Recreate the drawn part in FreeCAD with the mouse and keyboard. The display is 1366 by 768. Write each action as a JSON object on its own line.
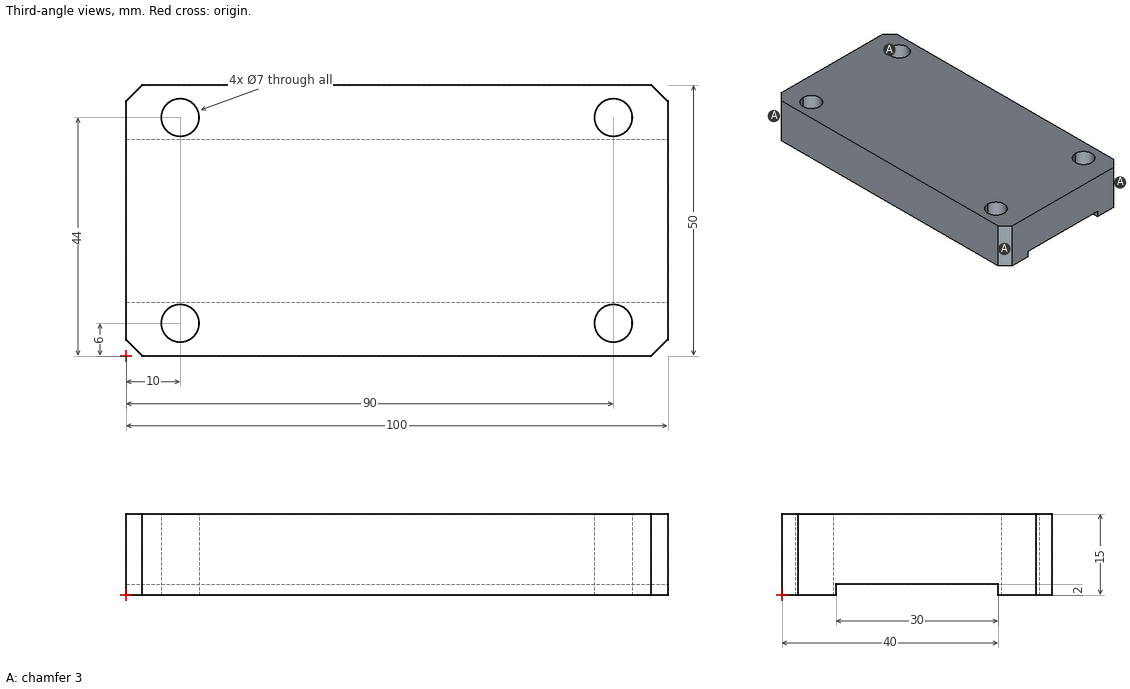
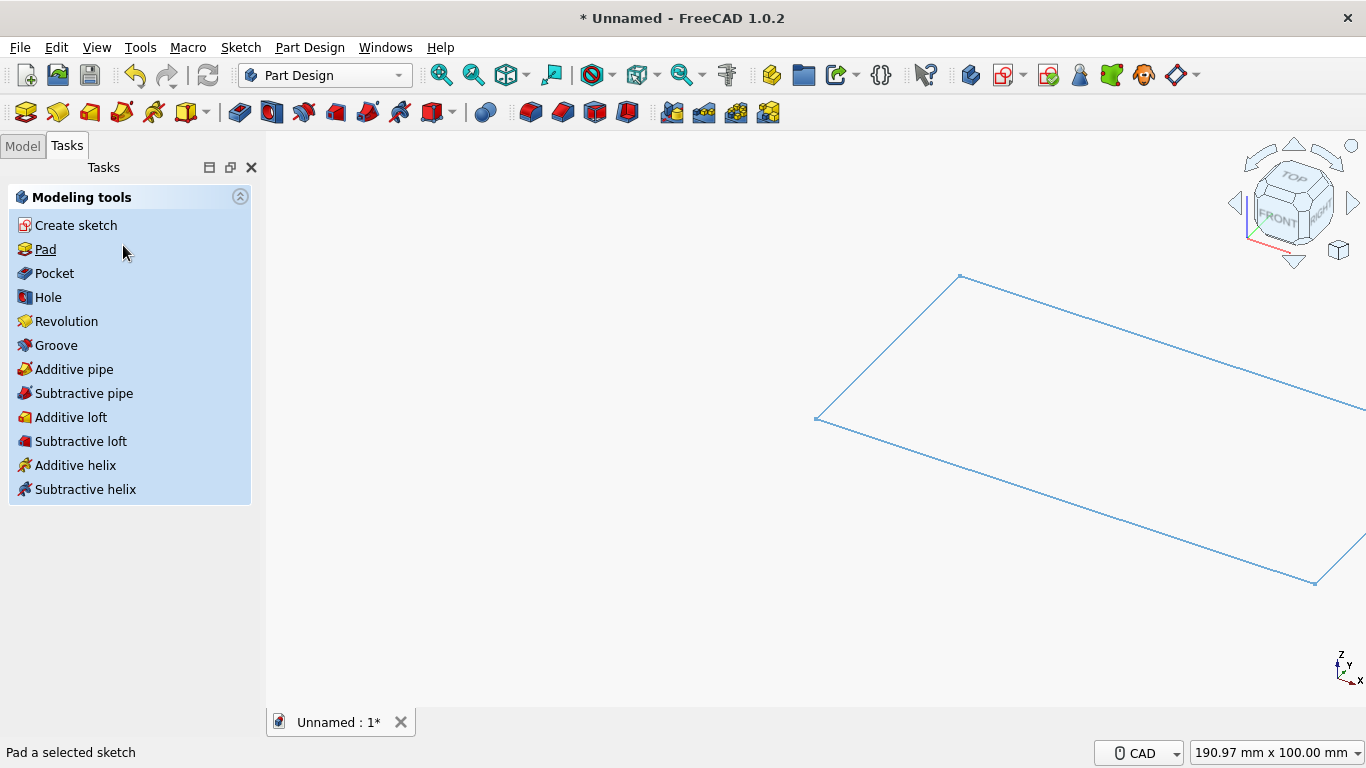
{"action": "left_click", "coordinate": [26, 112]}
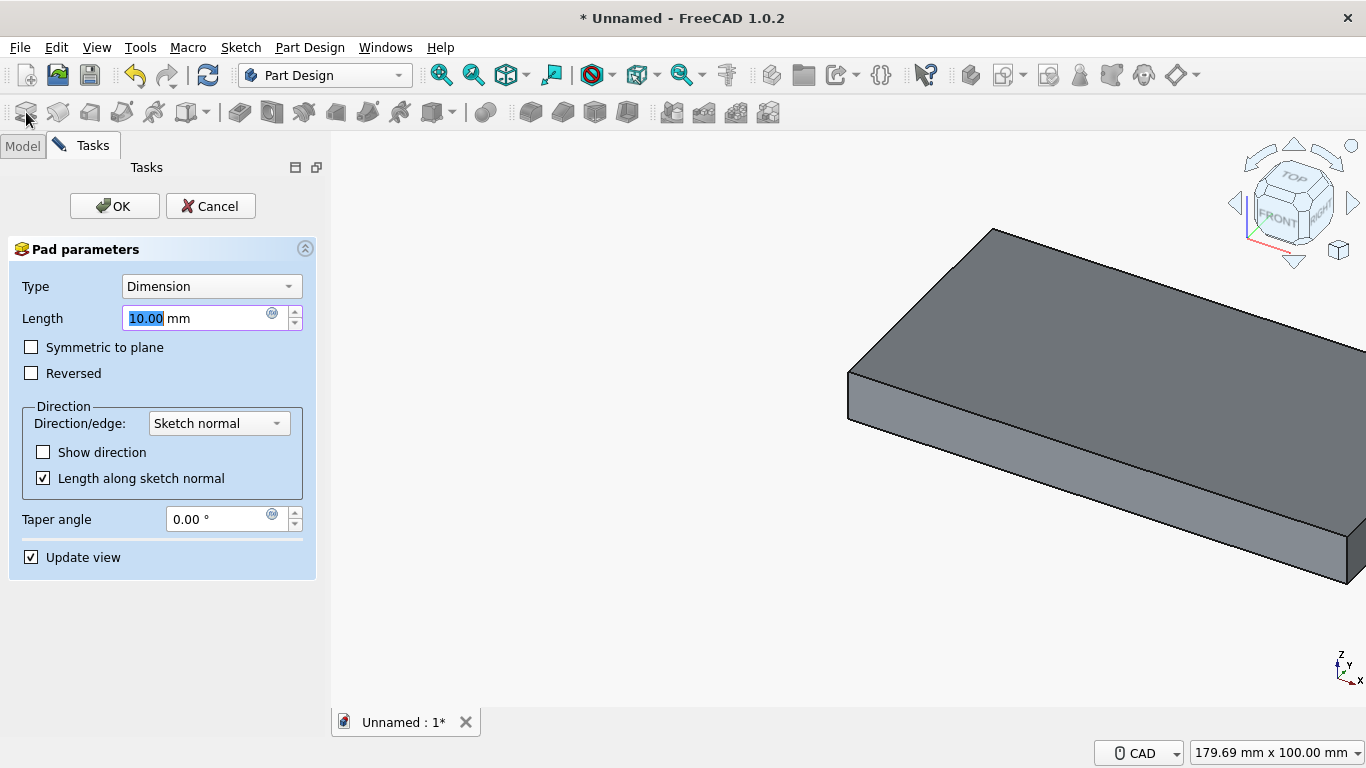
{"action": "type", "text": "15"}
{"action": "key", "text": "Tab"}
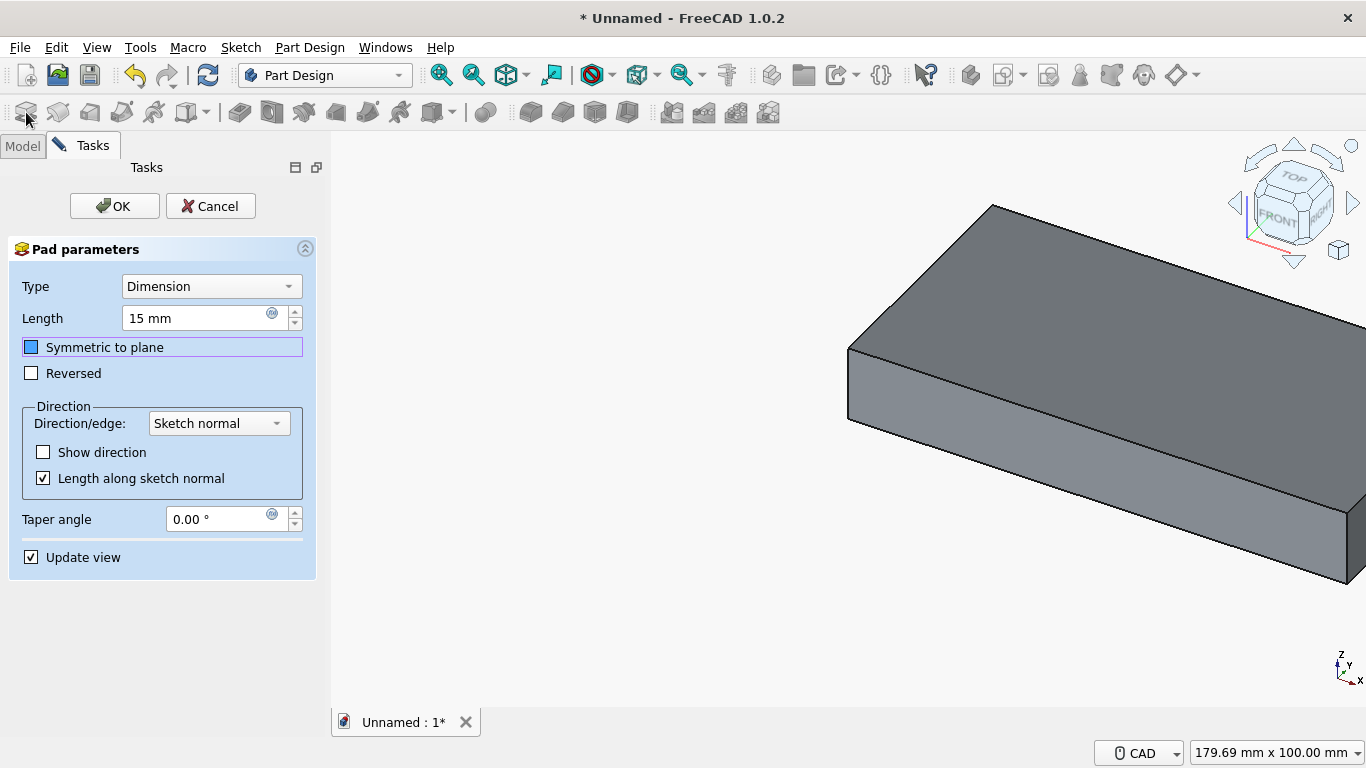
{"action": "left_click", "coordinate": [115, 206]}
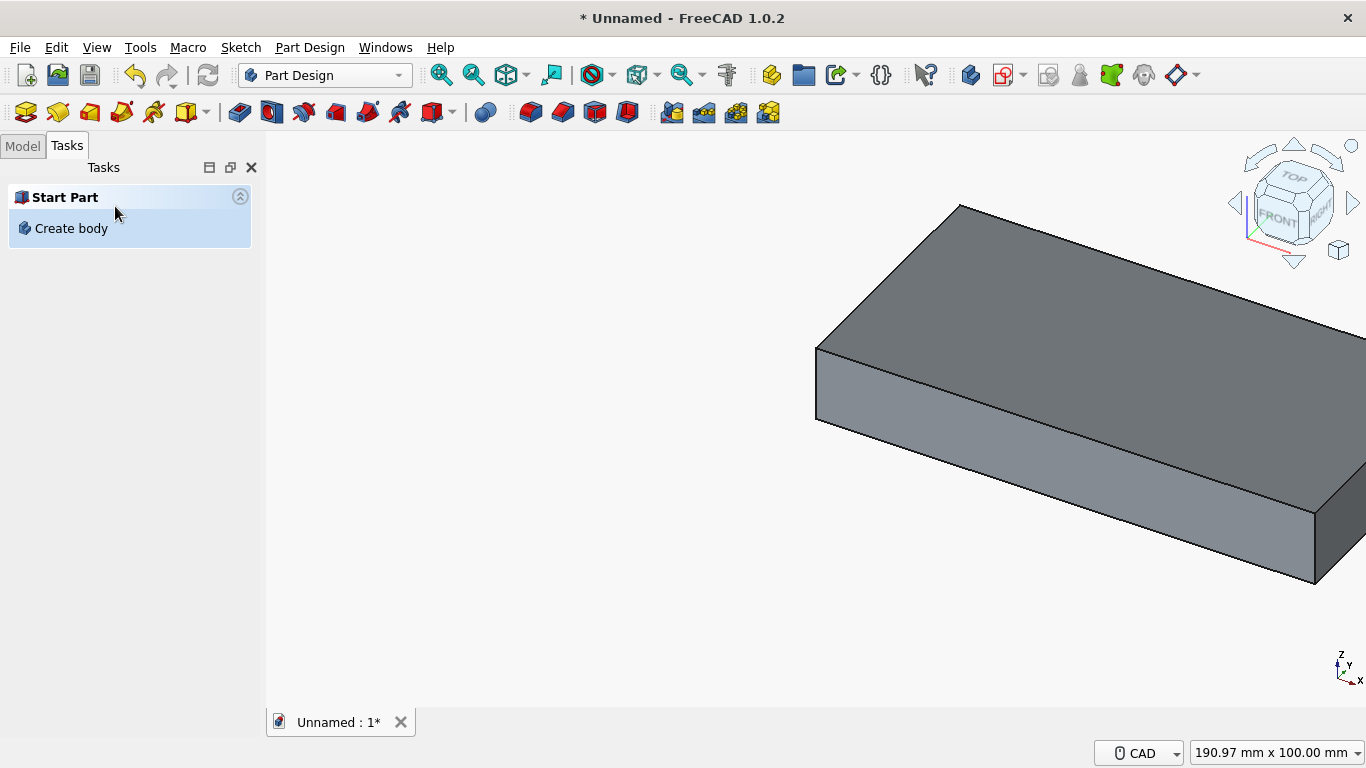
{"action": "key", "text": "v f"}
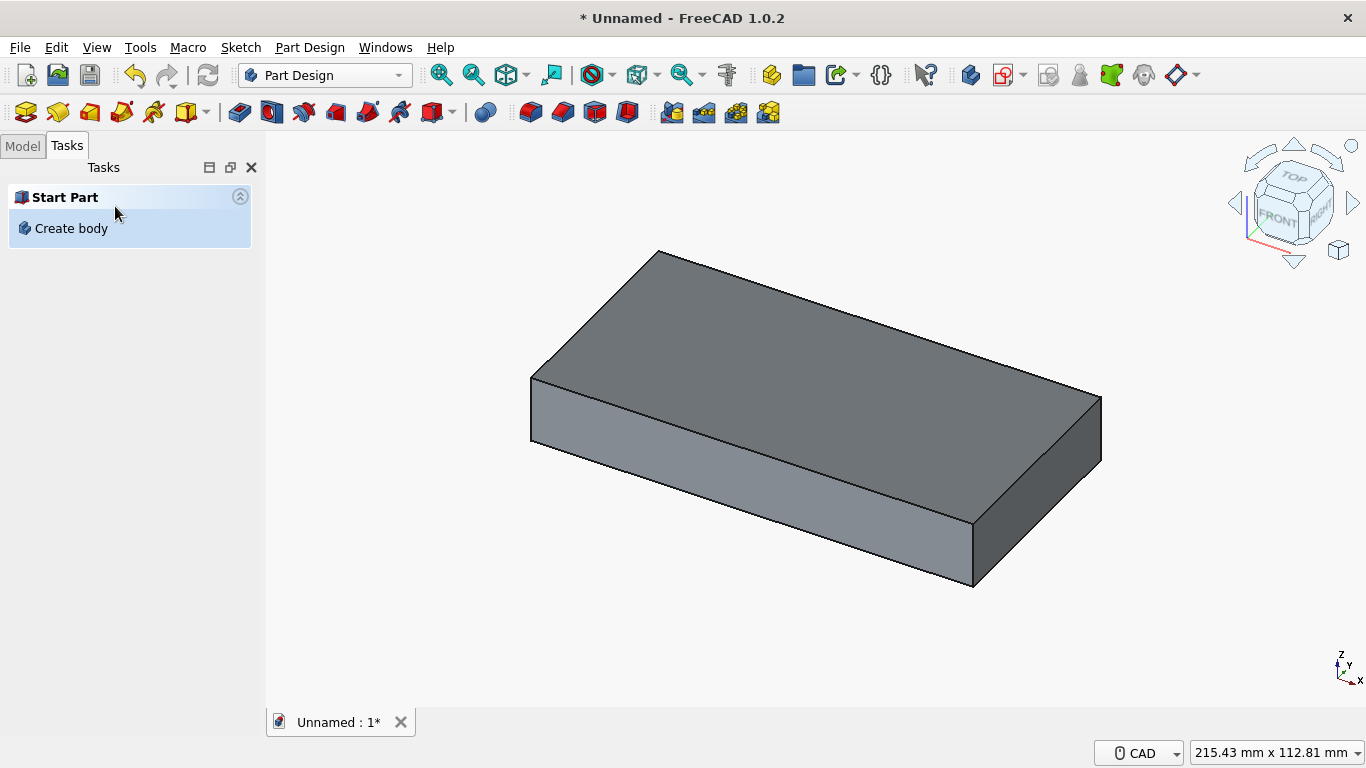
{"action": "key", "text": "5"}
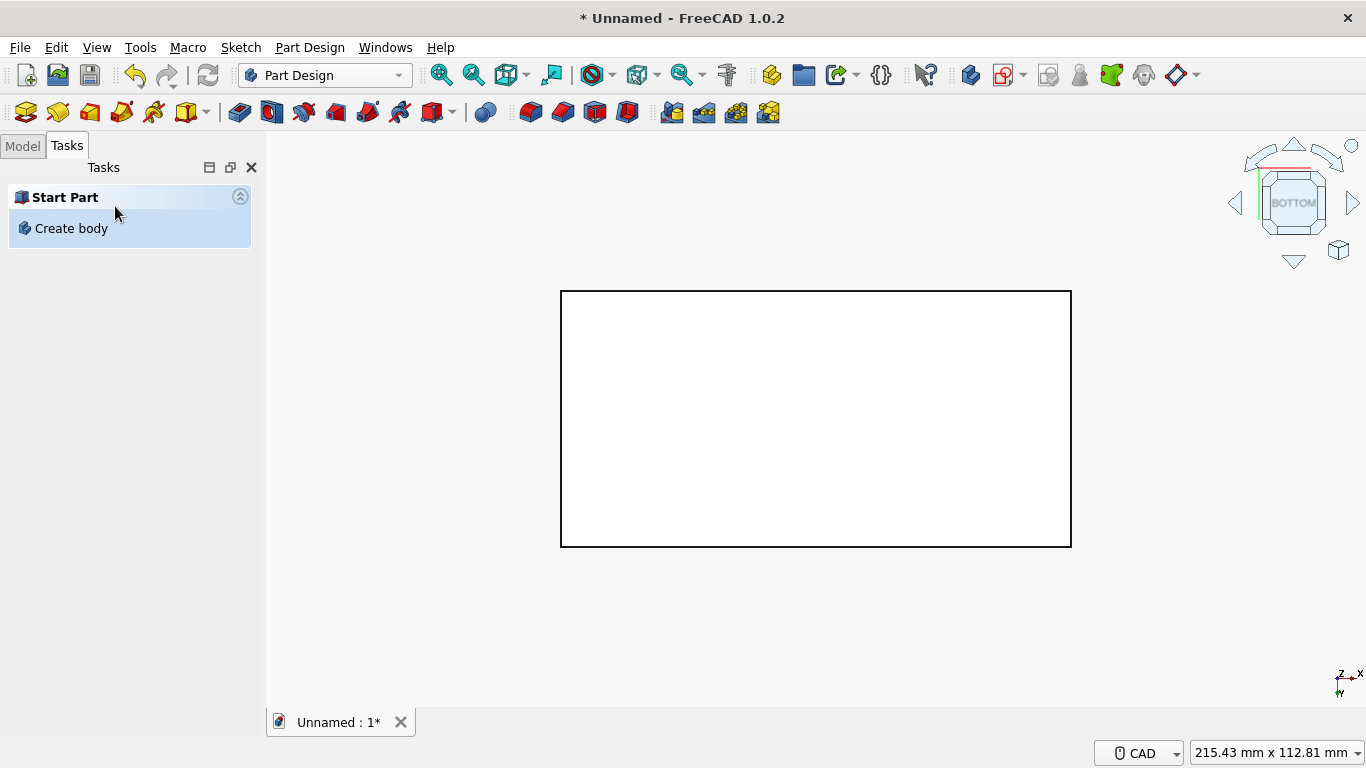
{"action": "left_click", "coordinate": [889, 418]}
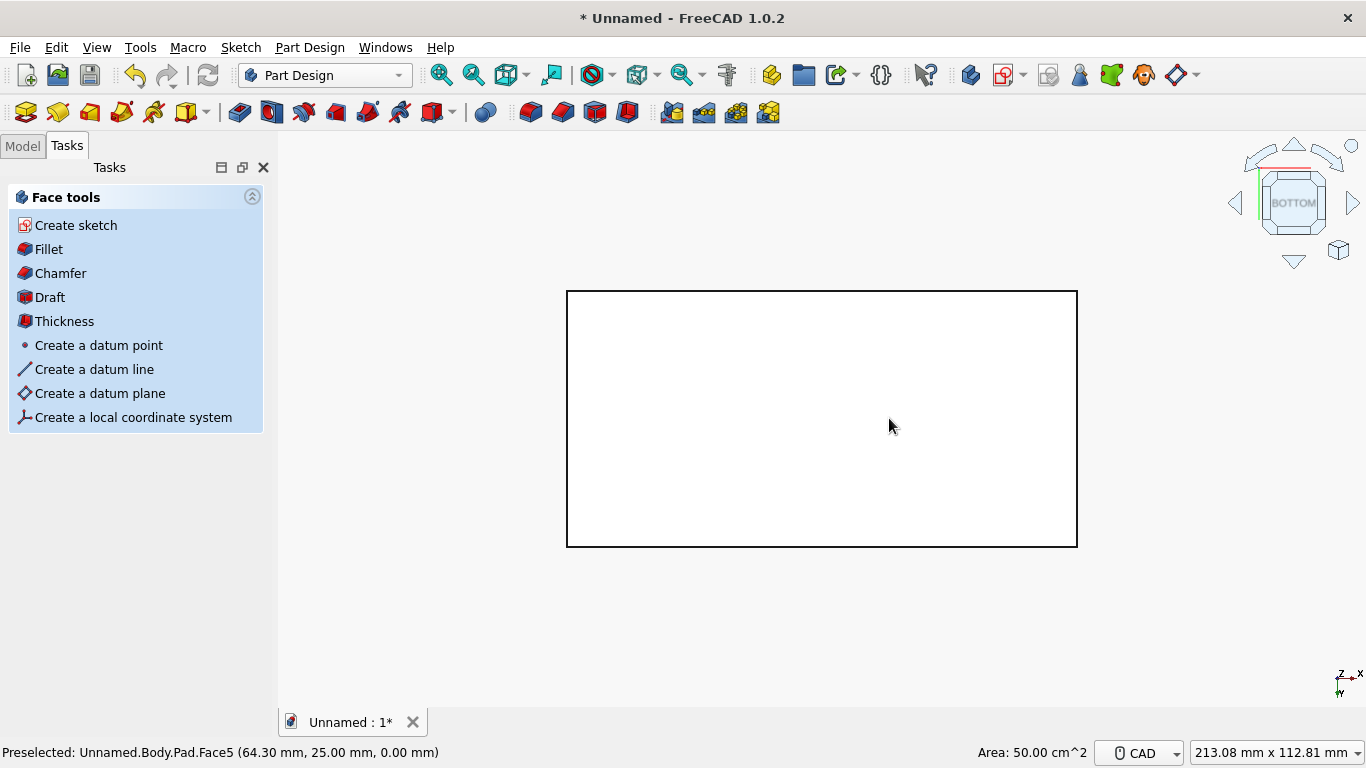
{"action": "left_click", "coordinate": [1004, 76]}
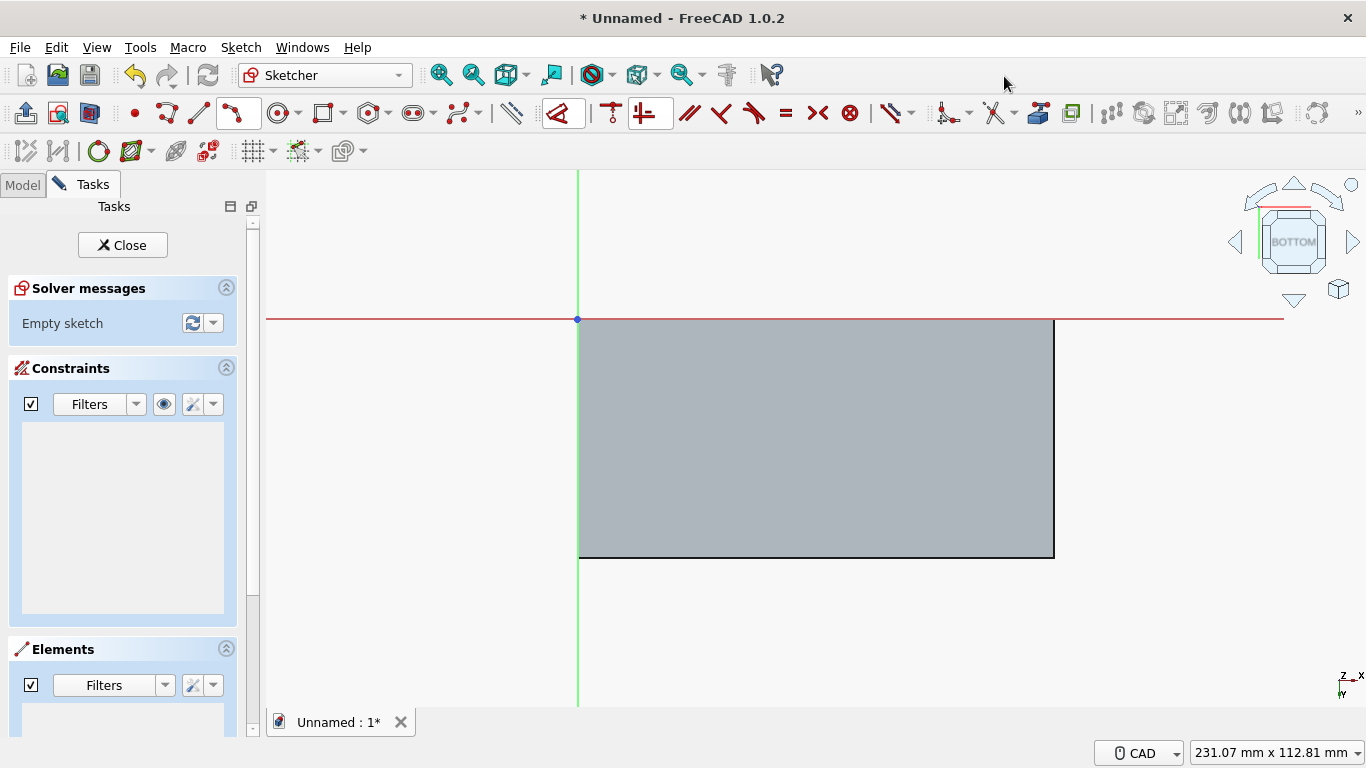
{"action": "scroll", "coordinate": [908, 420], "scroll_direction": "up", "scroll_amount": 2}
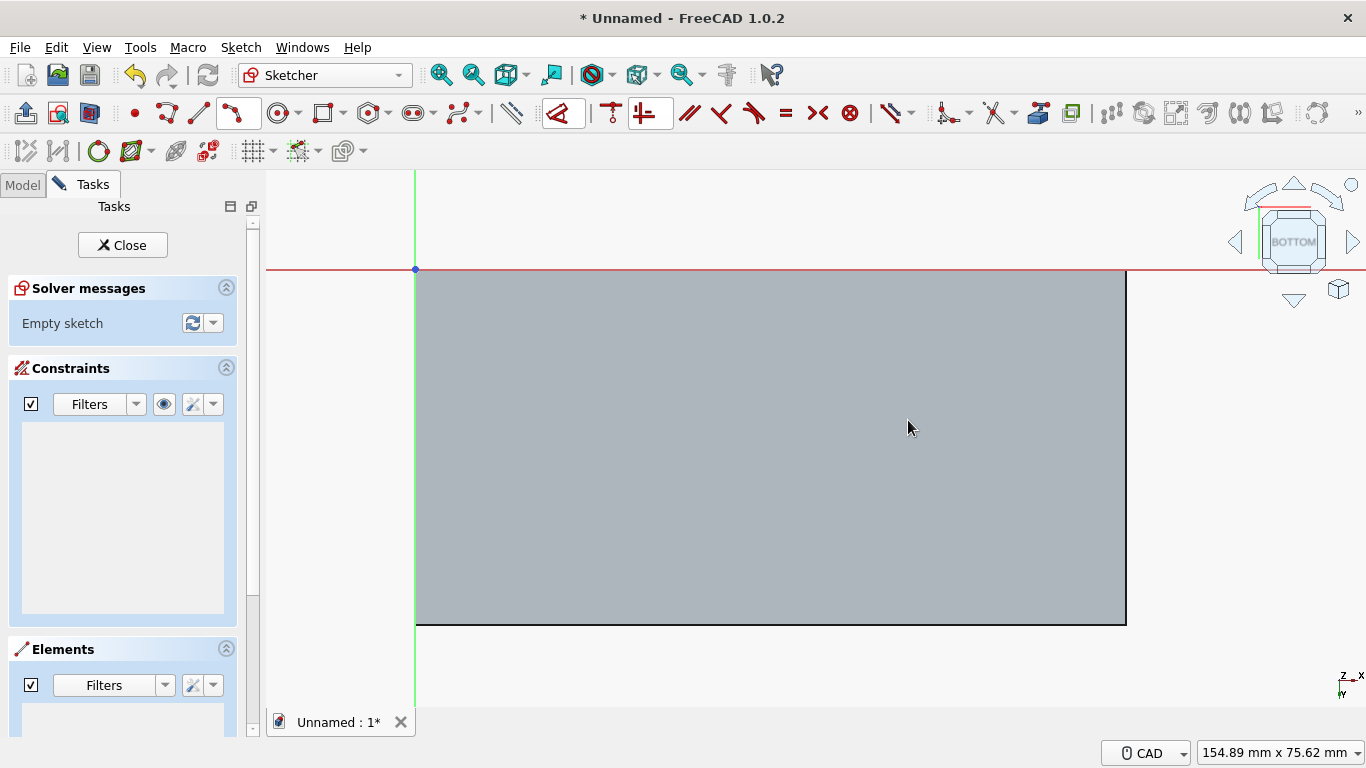
{"action": "key", "text": "g c"}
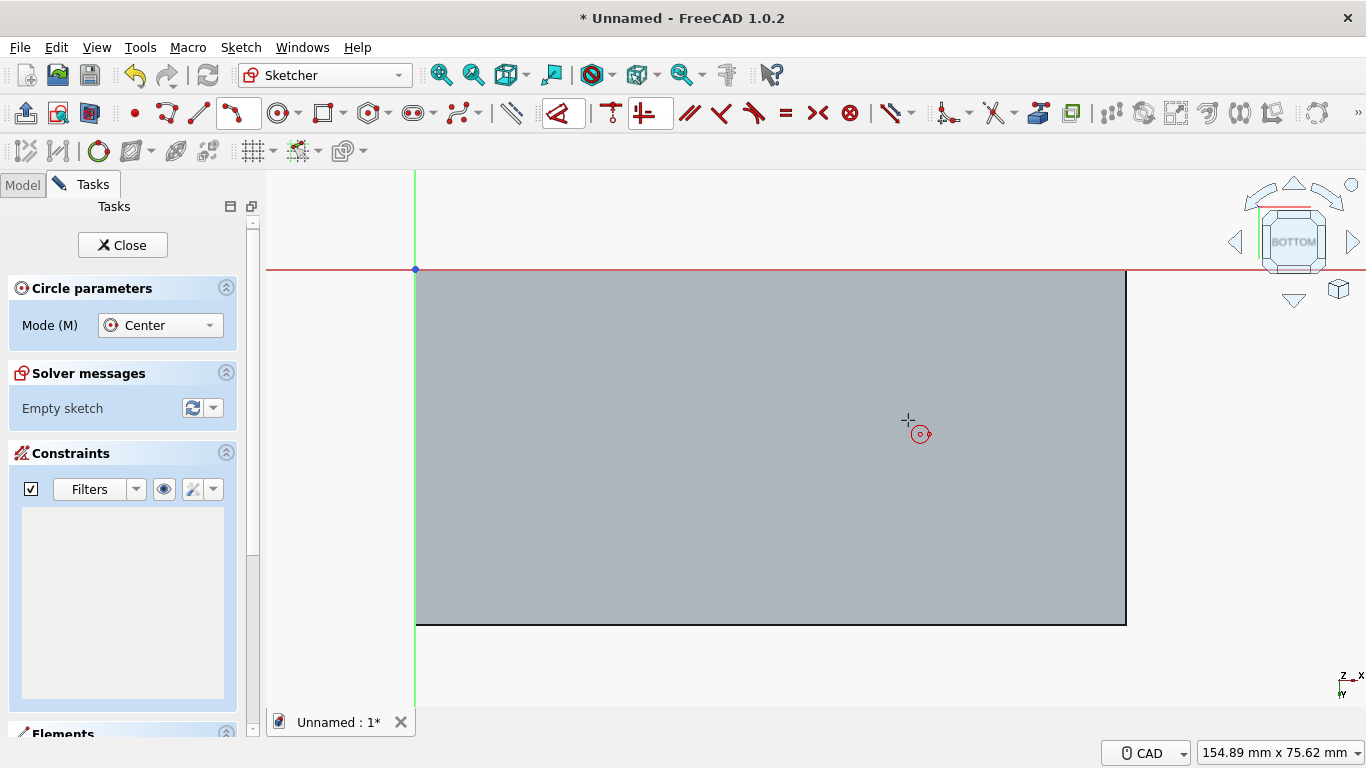
{"action": "left_click", "coordinate": [486, 582]}
{"action": "mouse_move", "coordinate": [504, 565]}